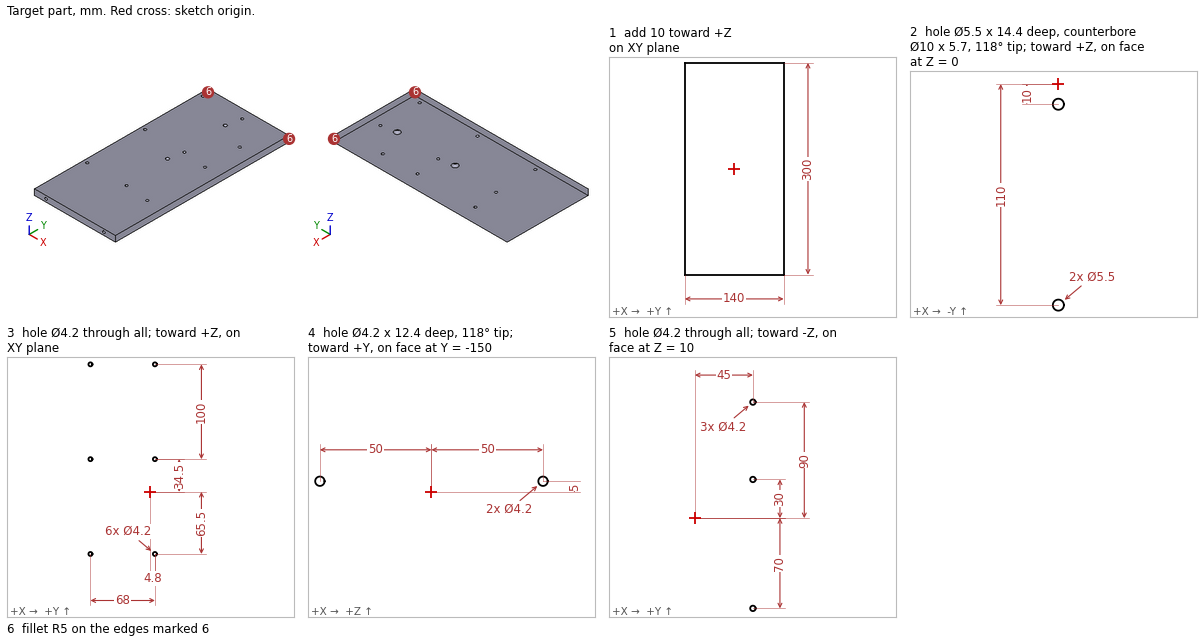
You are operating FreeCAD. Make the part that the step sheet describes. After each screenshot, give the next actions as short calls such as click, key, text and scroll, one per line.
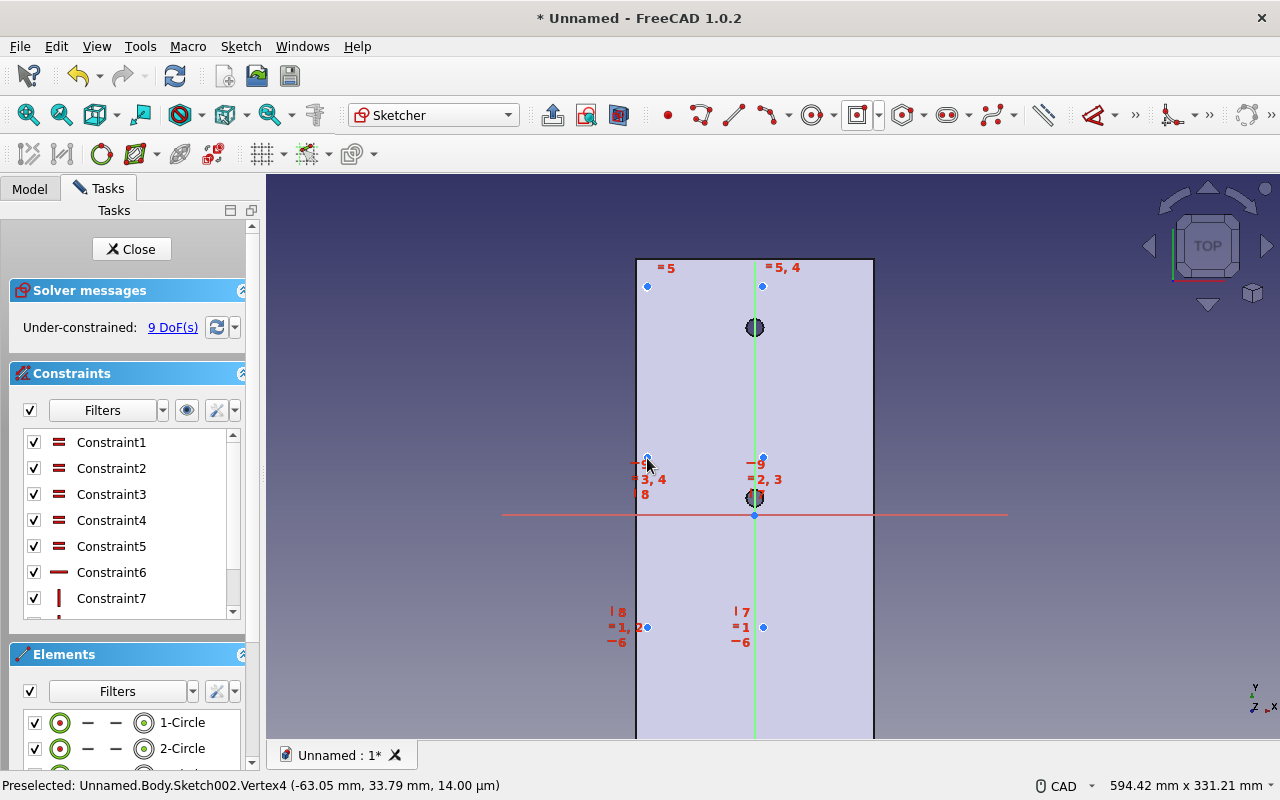
click(763, 457)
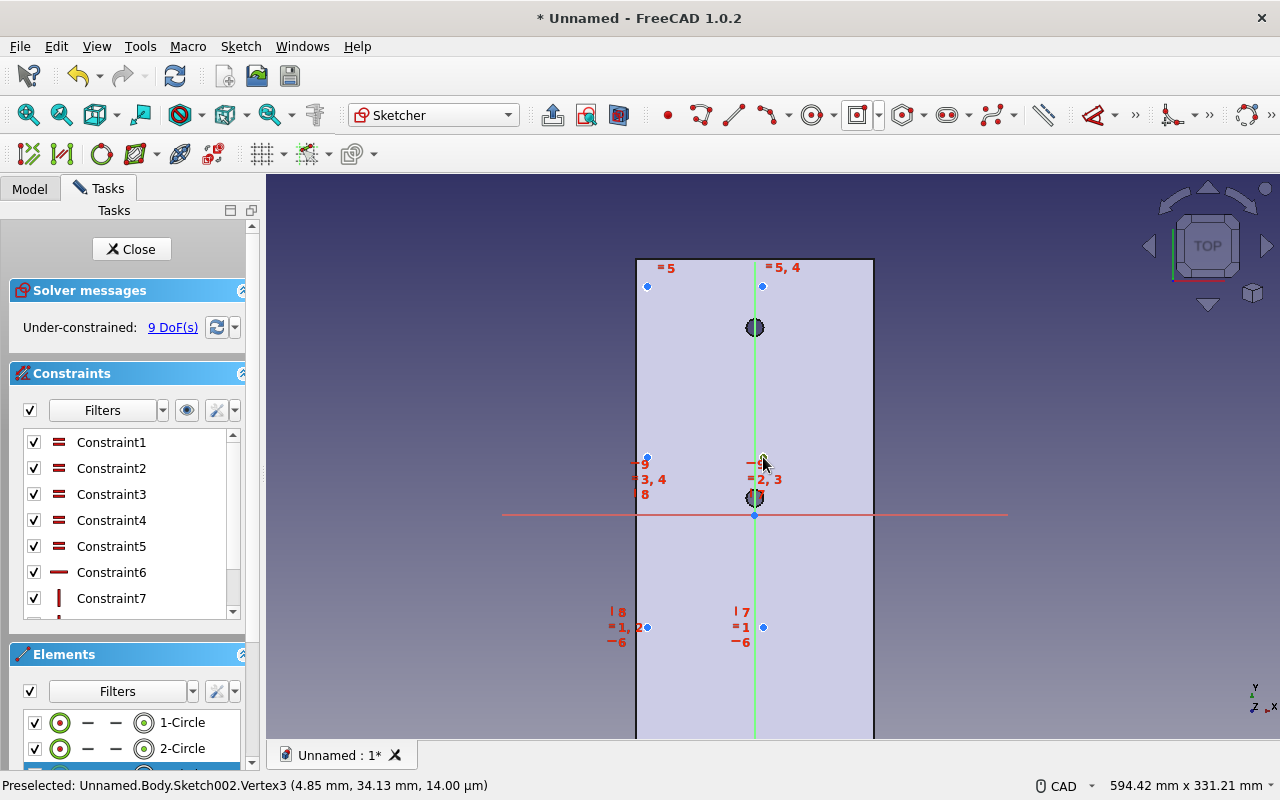
click(763, 286)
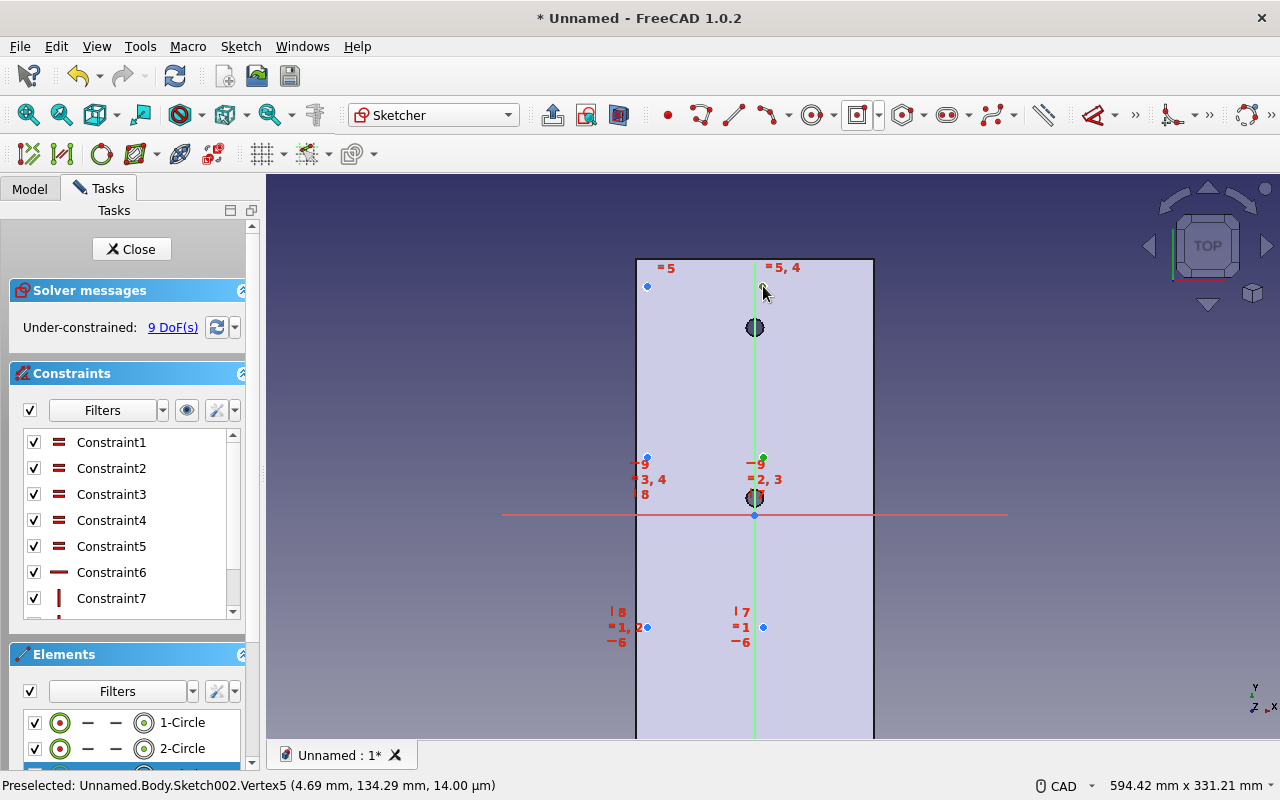
key(v)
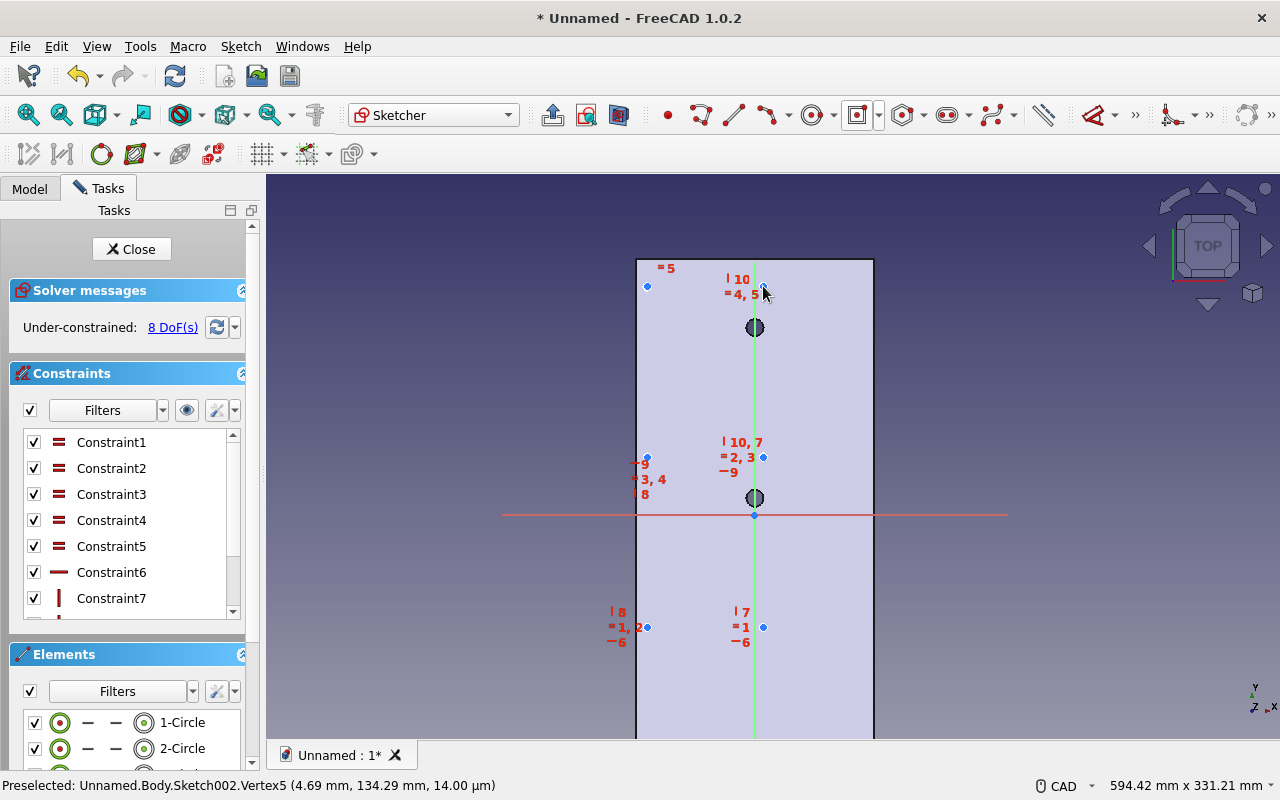
click(645, 455)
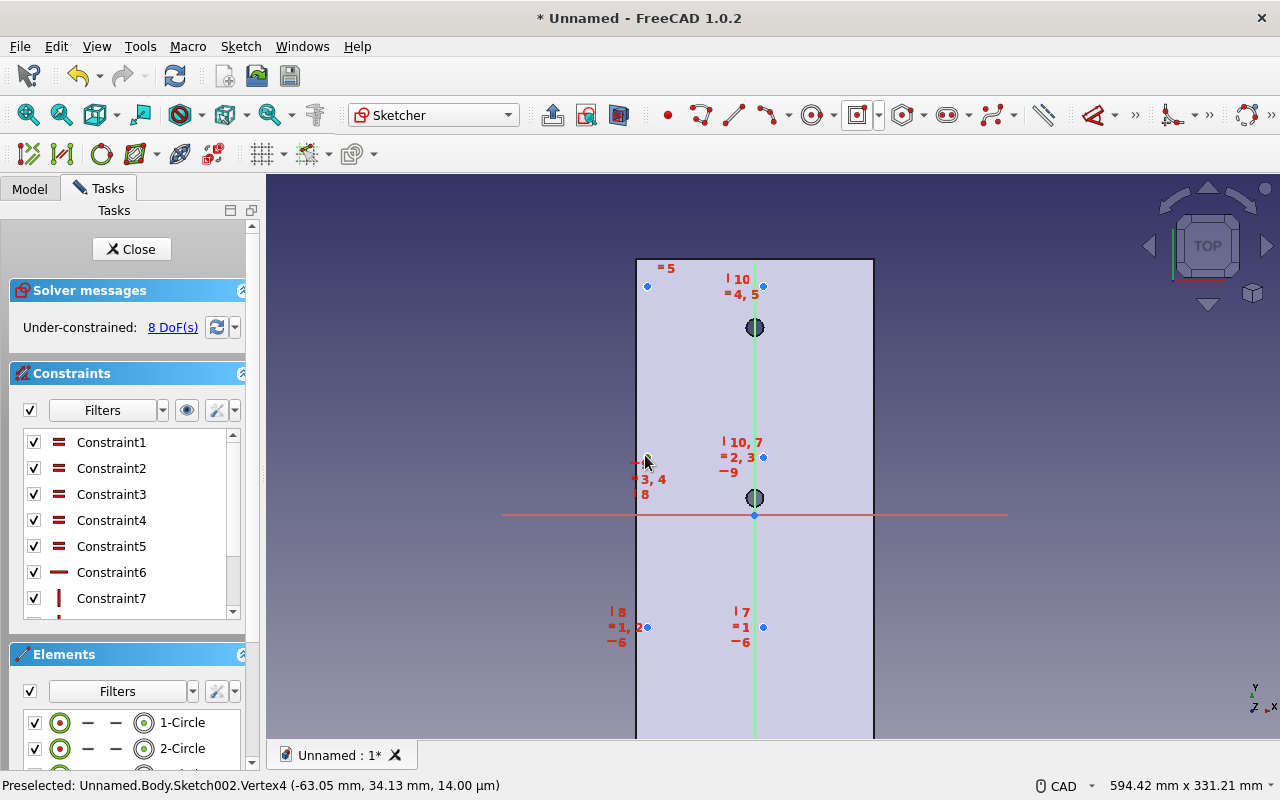
click(647, 287)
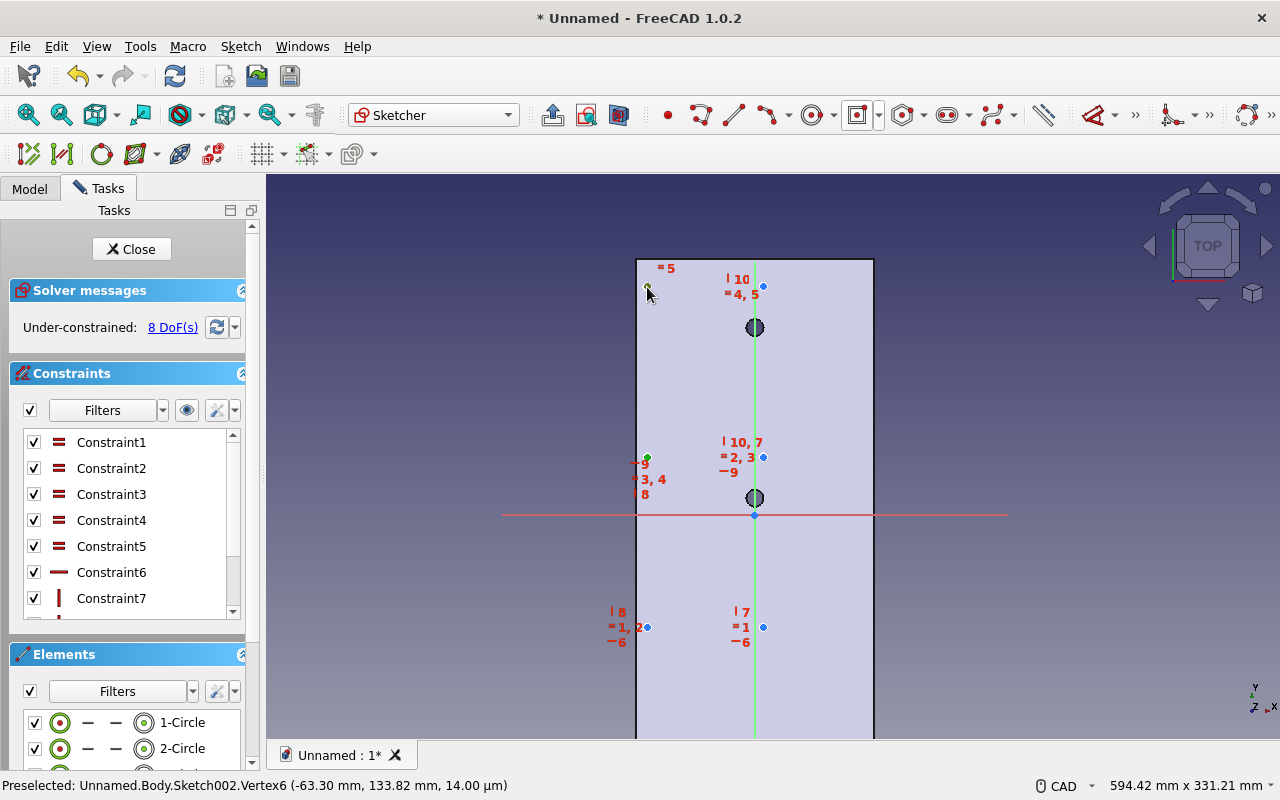
key(v)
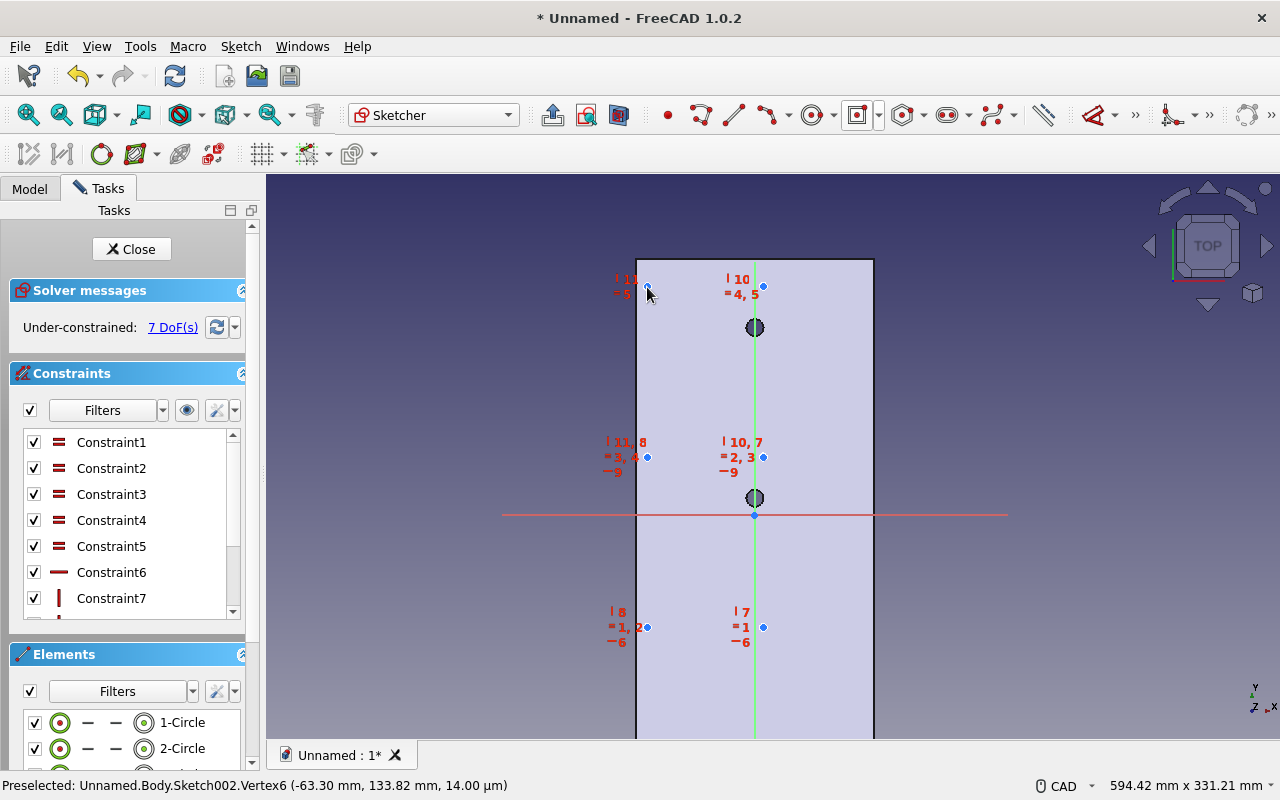
click(763, 286)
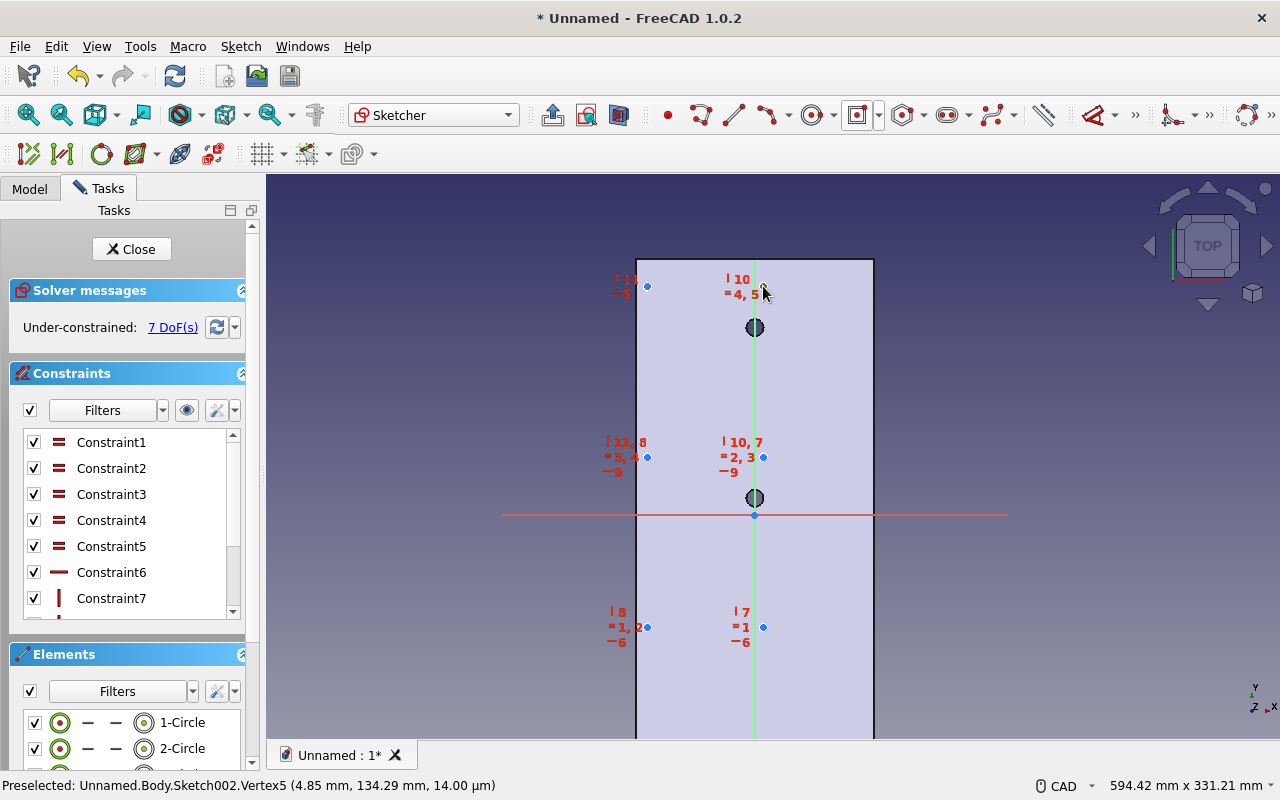
click(647, 287)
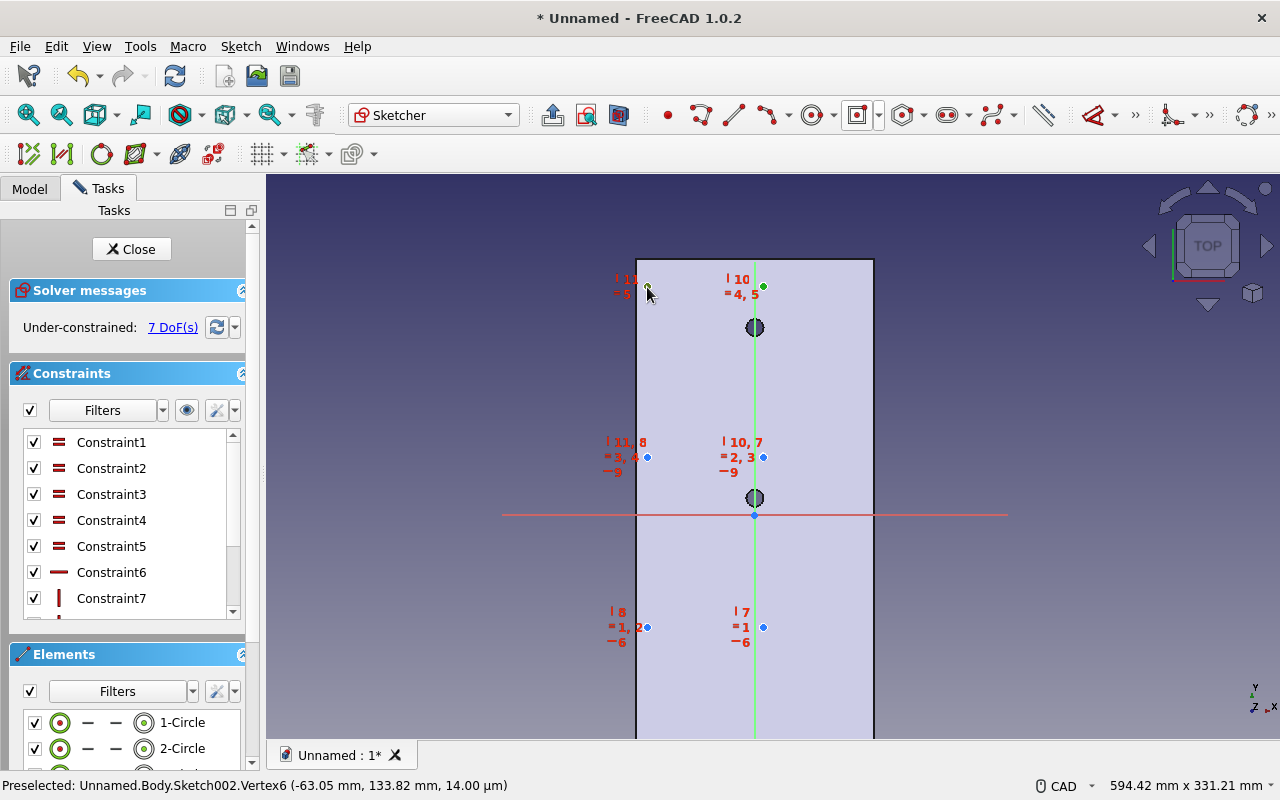
key(h)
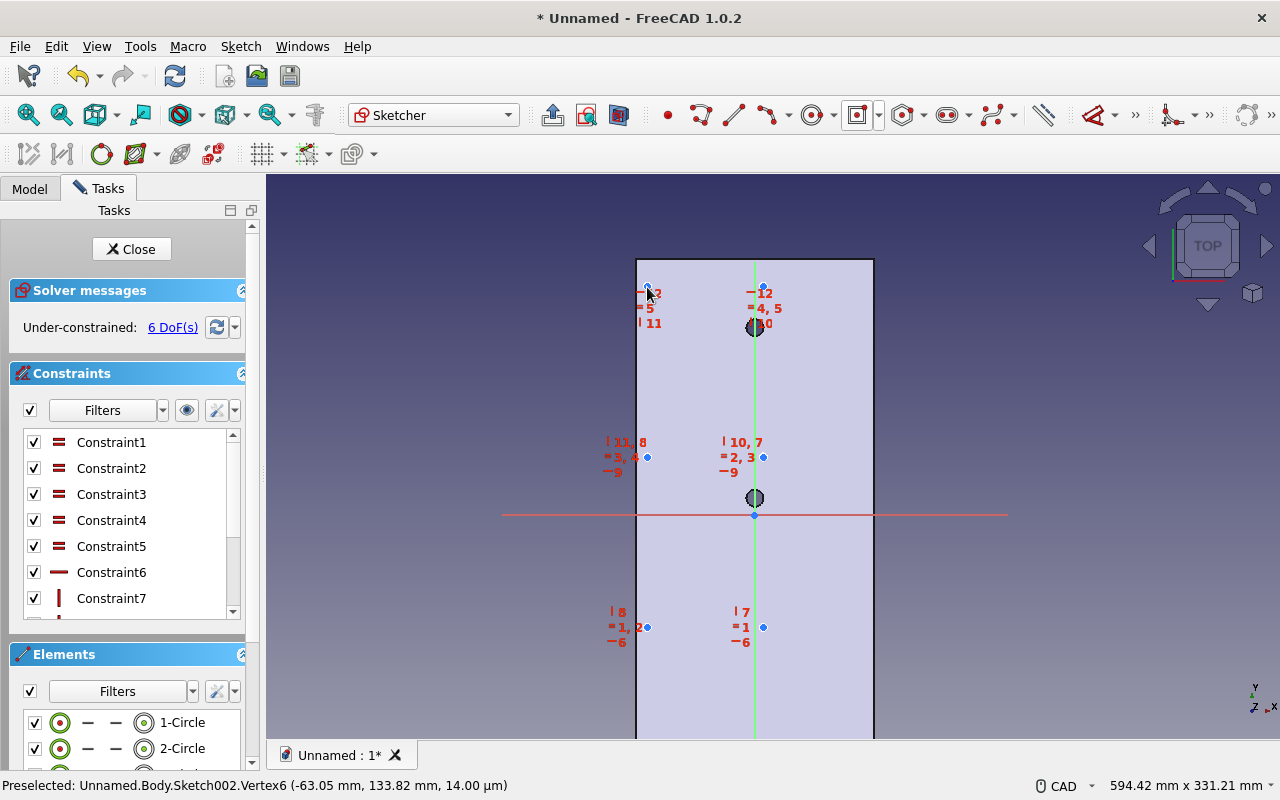
click(1092, 116)